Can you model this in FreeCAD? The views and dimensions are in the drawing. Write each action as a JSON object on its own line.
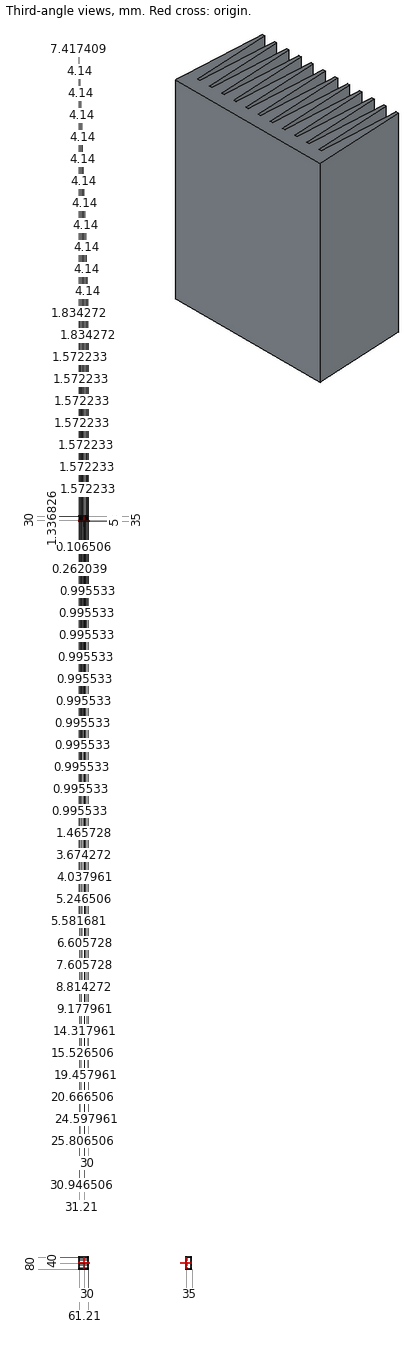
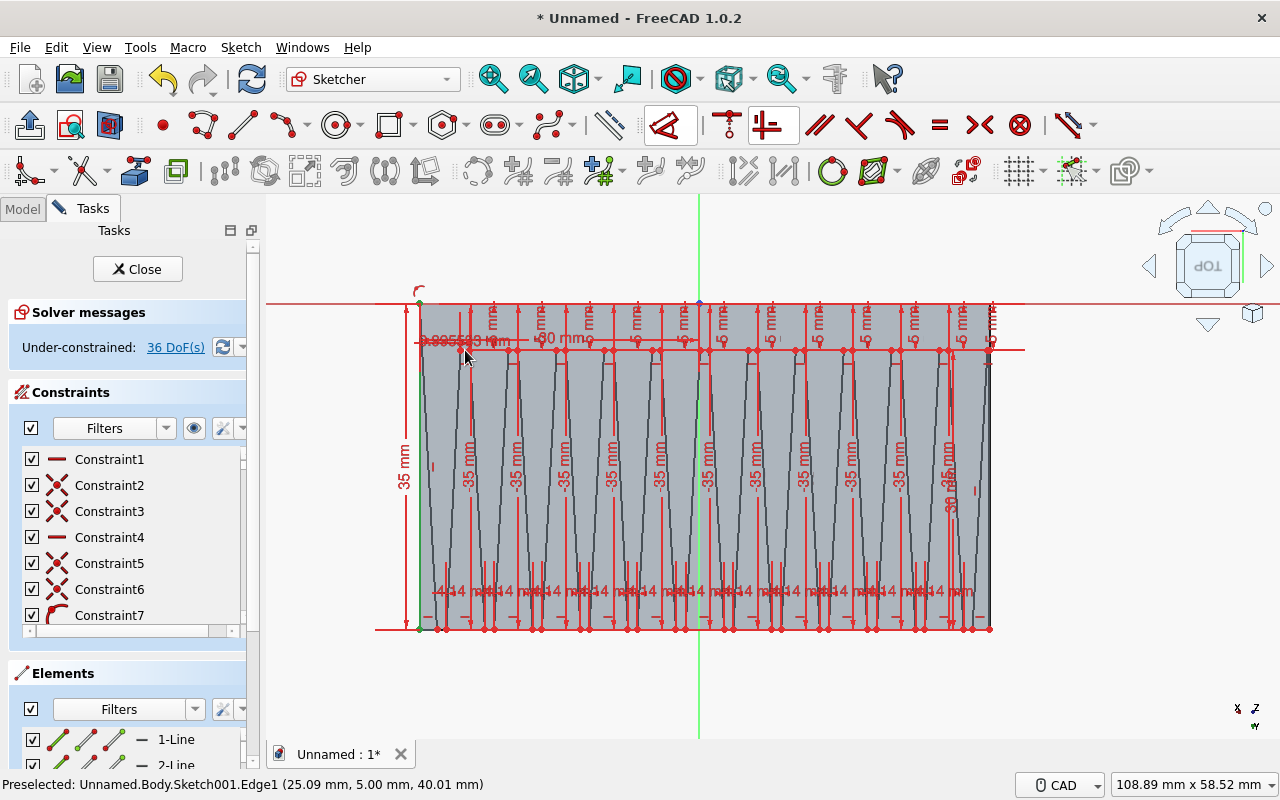
{"action": "scroll", "coordinate": [425, 630], "scroll_direction": "up", "scroll_amount": 5}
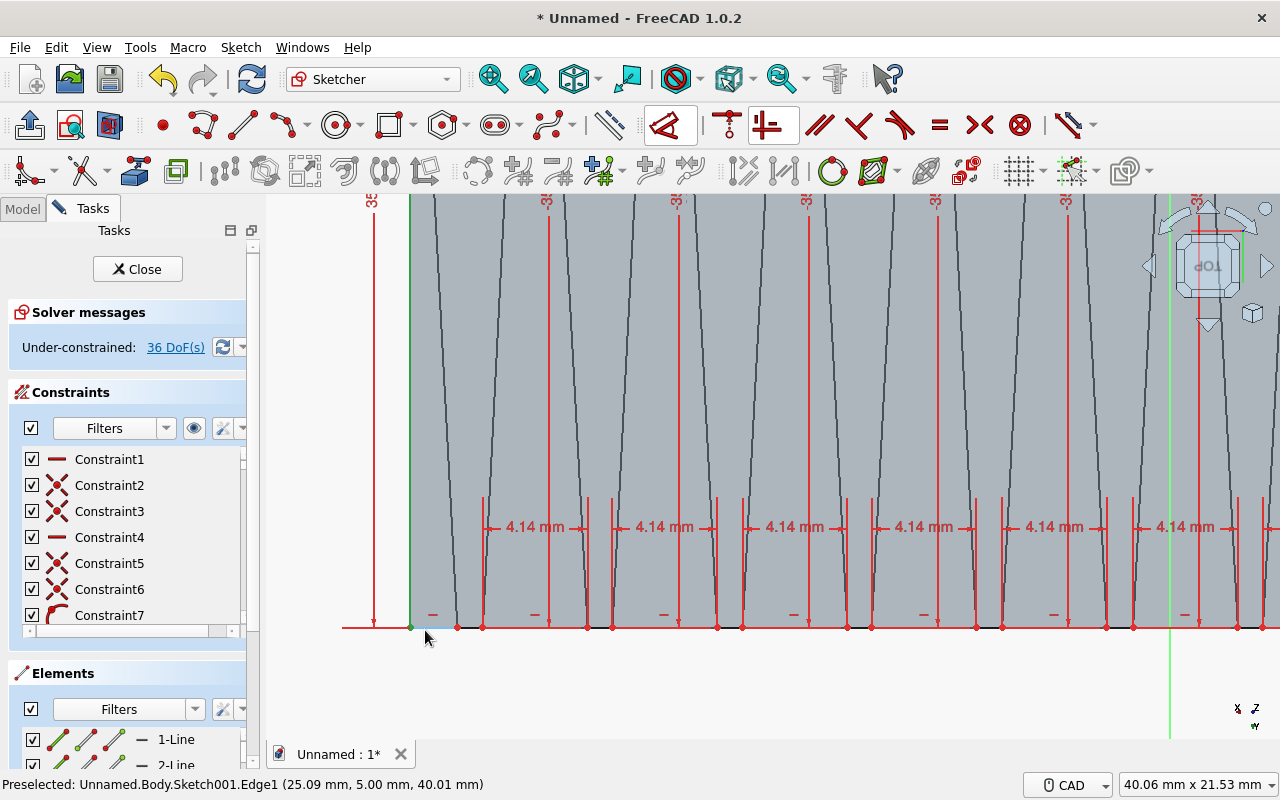
{"action": "left_click", "coordinate": [424, 628]}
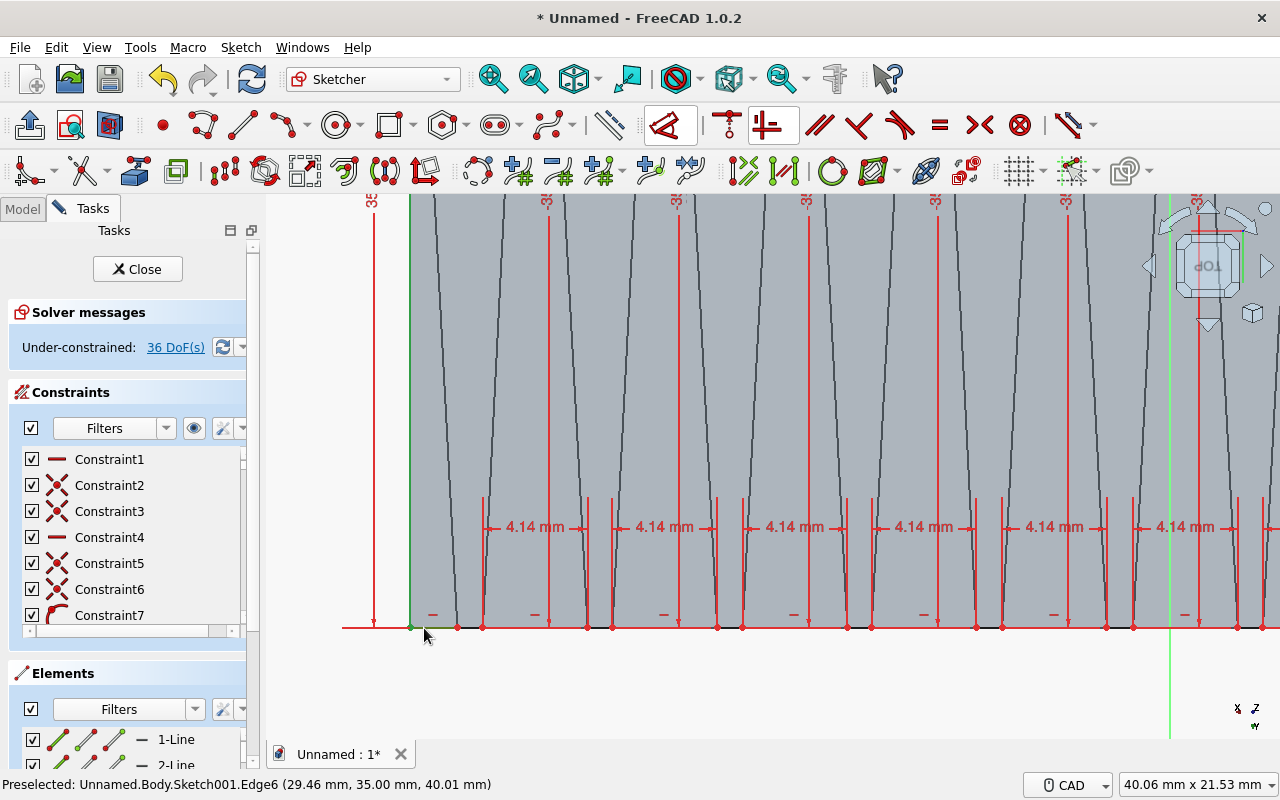
{"action": "left_click", "coordinate": [692, 126]}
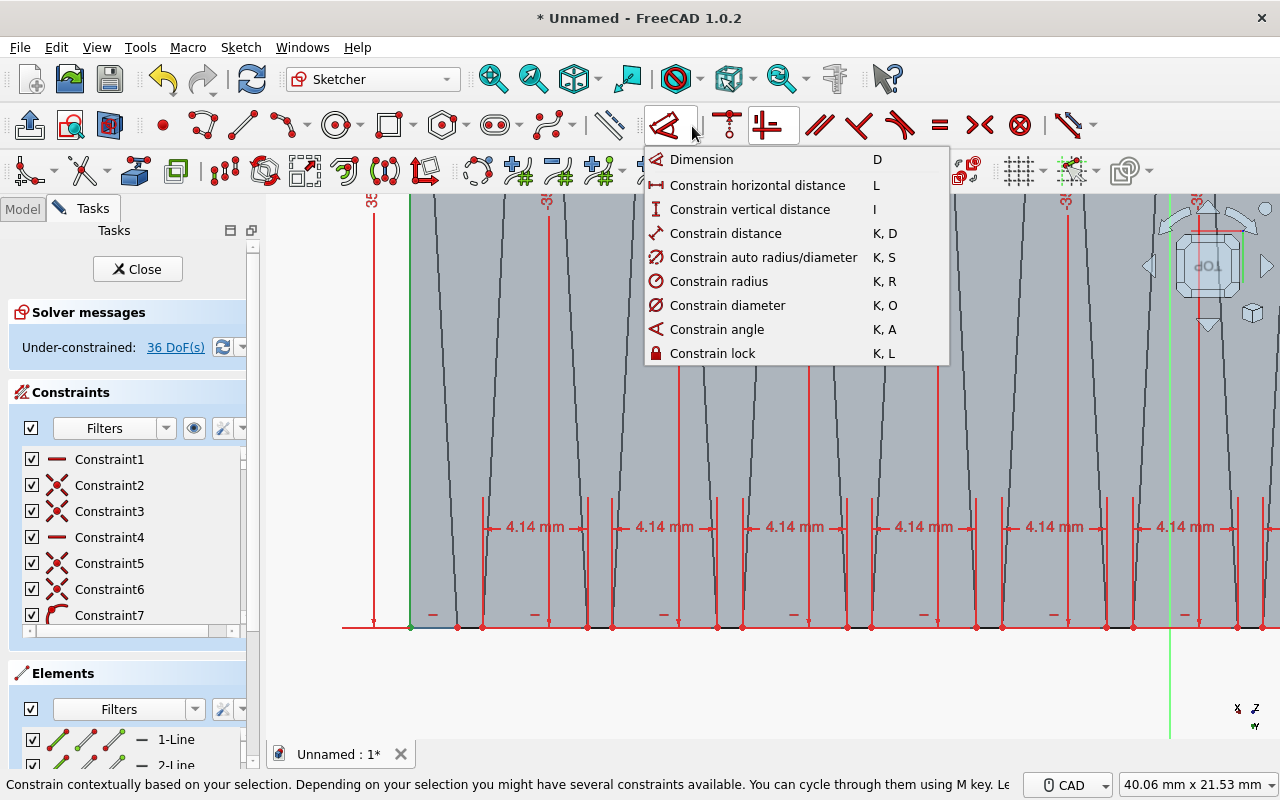
{"action": "left_click", "coordinate": [797, 185]}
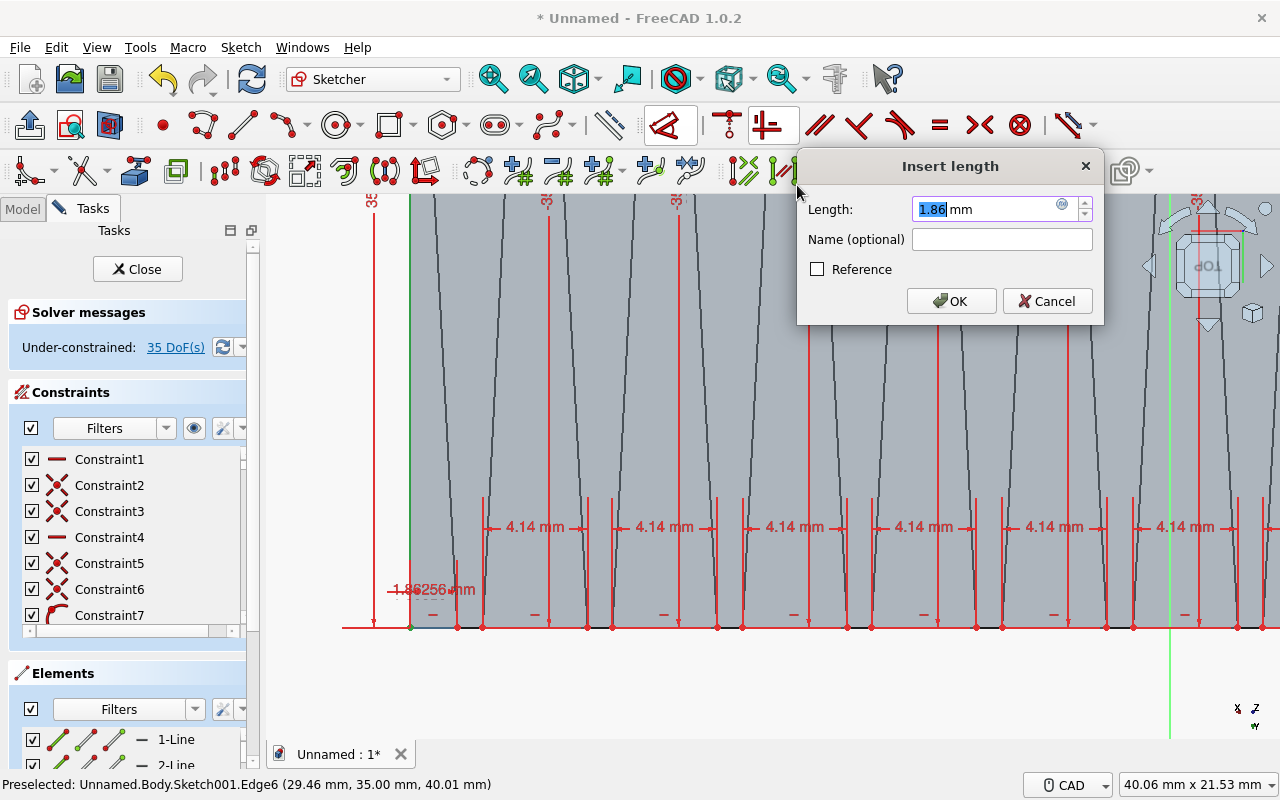
{"action": "type", "text": "1.834272"}
{"action": "key", "text": "Return"}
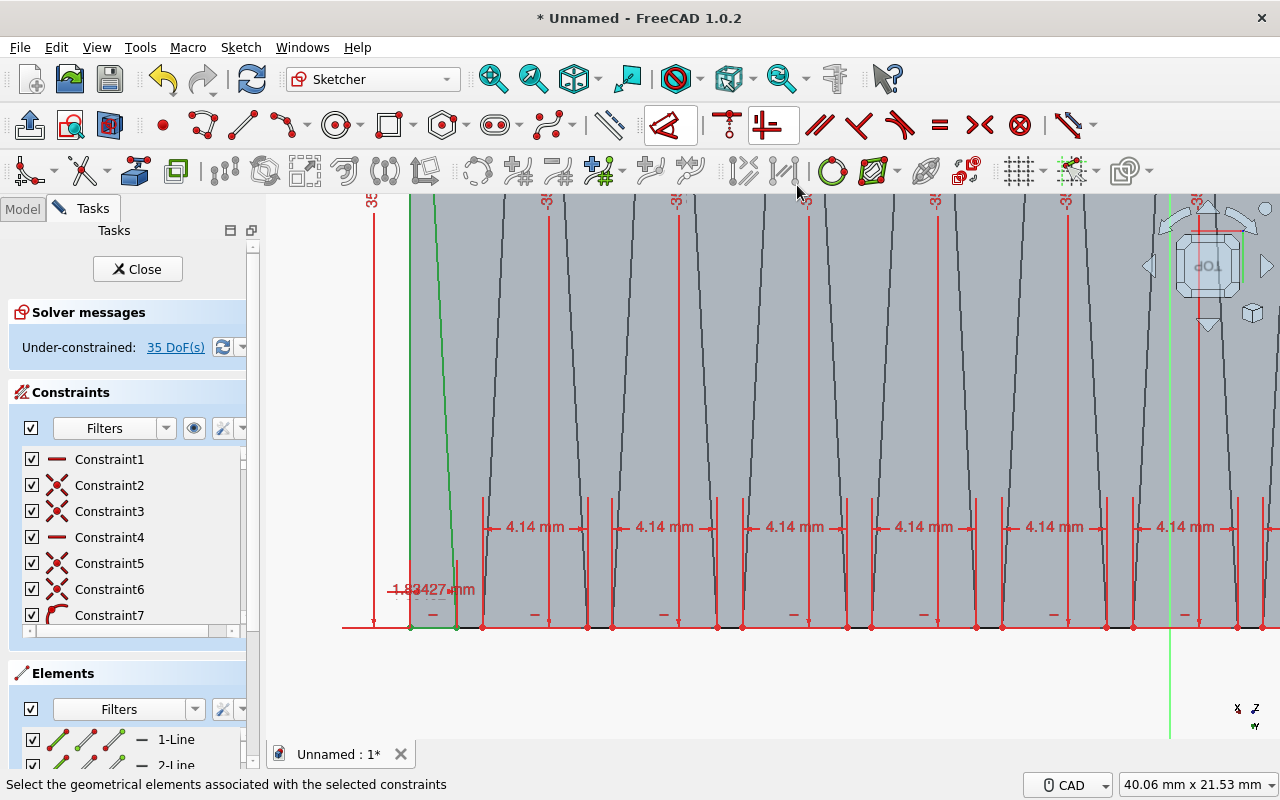
{"action": "scroll", "coordinate": [425, 630], "scroll_direction": "down", "scroll_amount": 5}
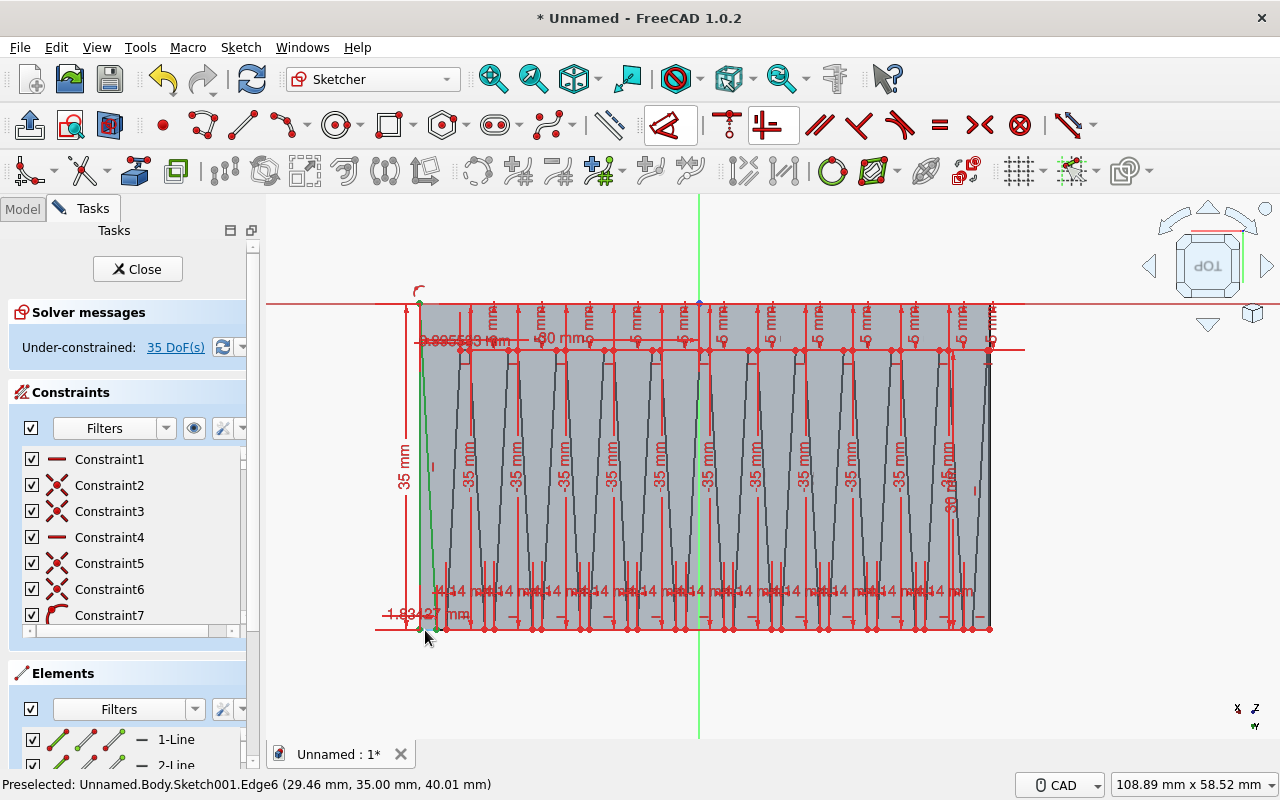
{"action": "scroll", "coordinate": [514, 350], "scroll_direction": "up", "scroll_amount": 8}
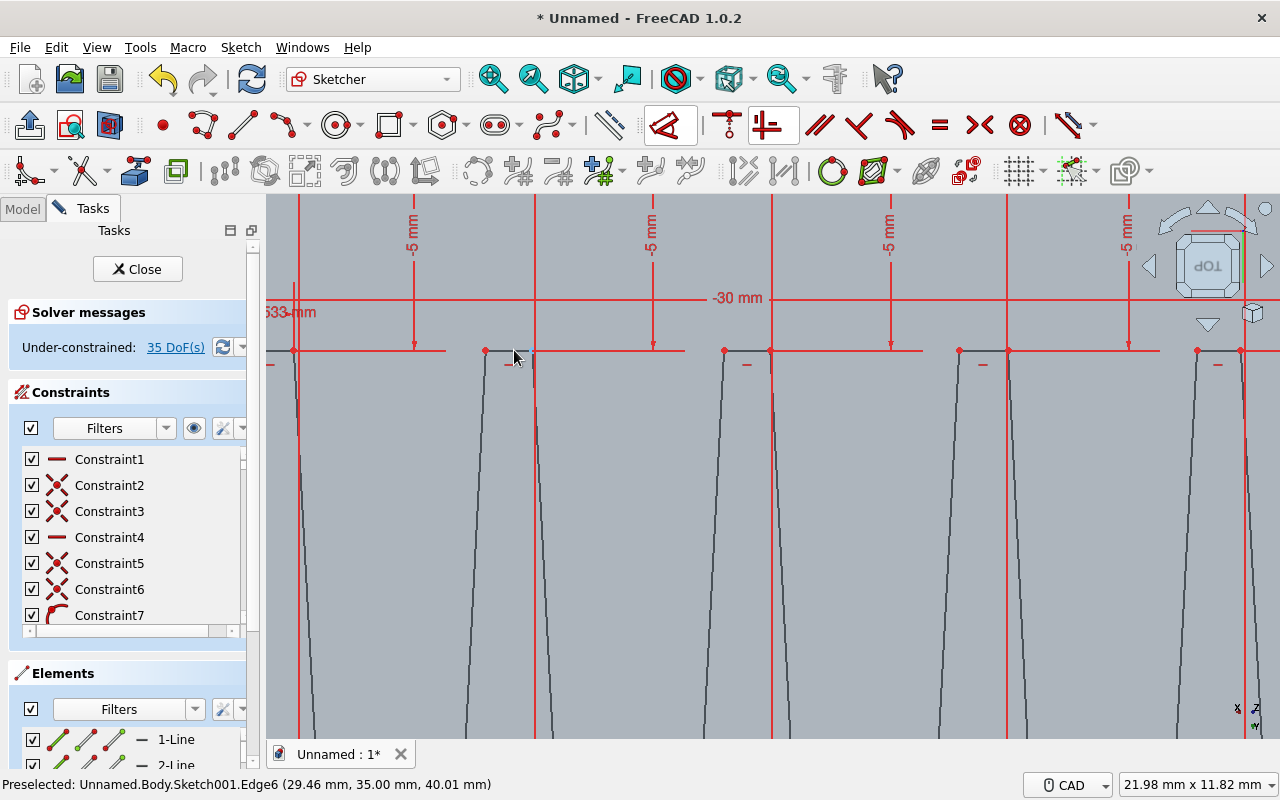
{"action": "left_click", "coordinate": [514, 351]}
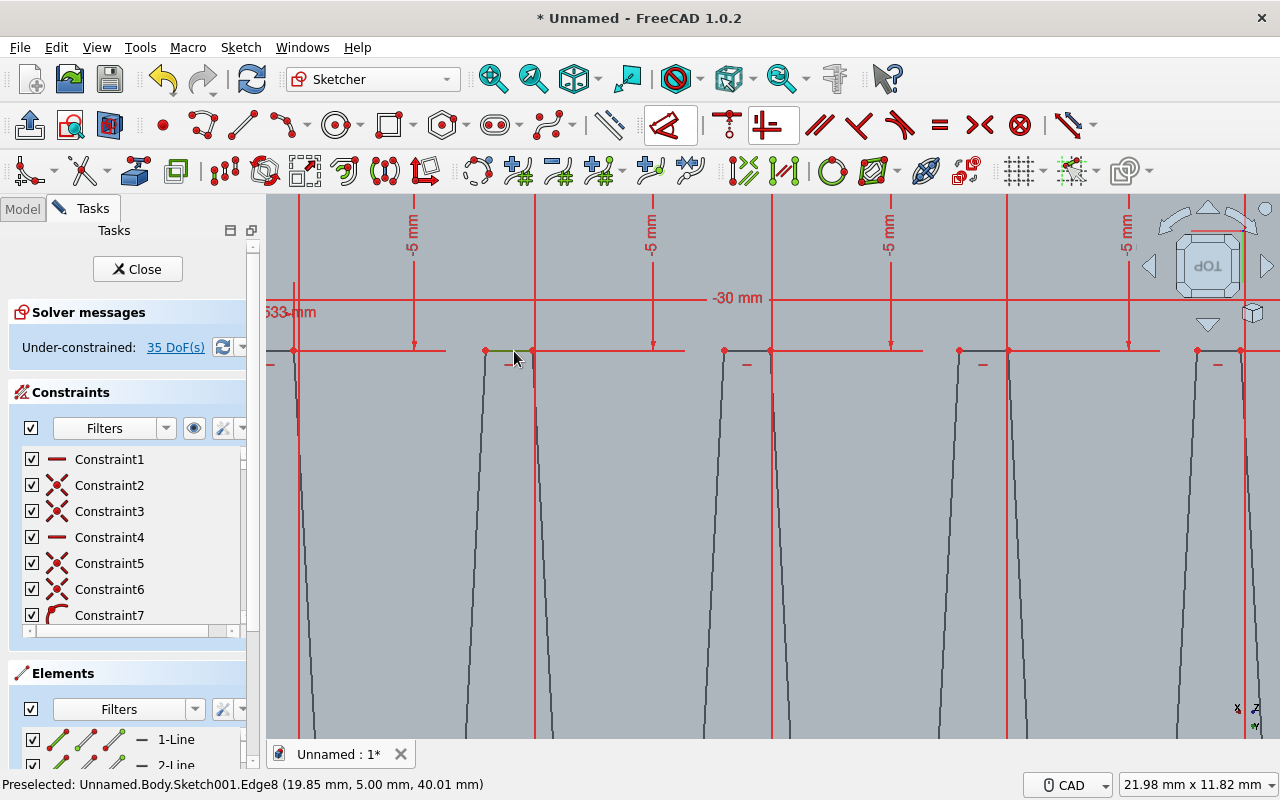
{"action": "left_click", "coordinate": [692, 126]}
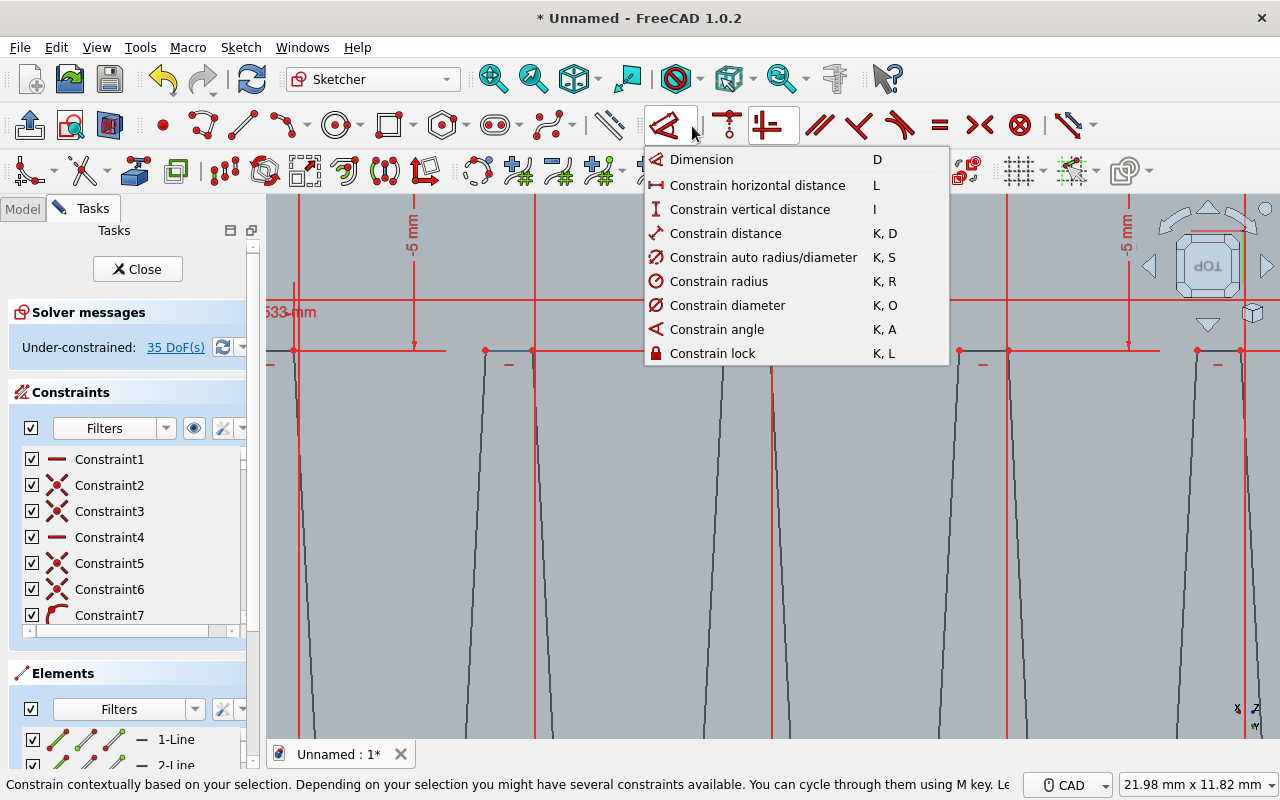
{"action": "left_click", "coordinate": [797, 185]}